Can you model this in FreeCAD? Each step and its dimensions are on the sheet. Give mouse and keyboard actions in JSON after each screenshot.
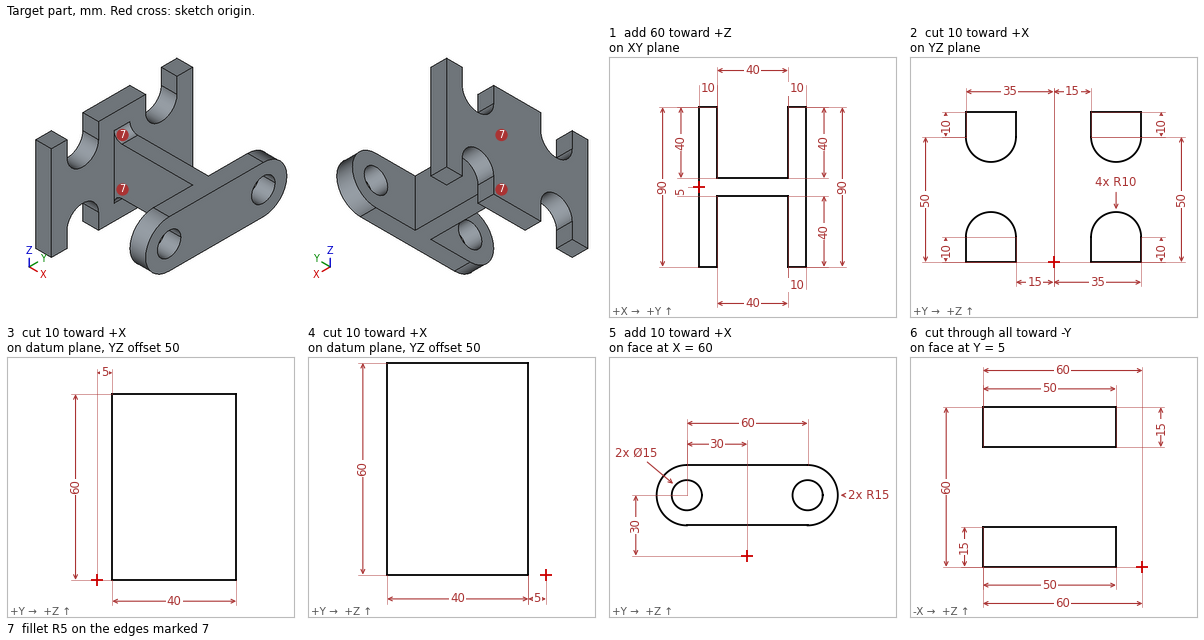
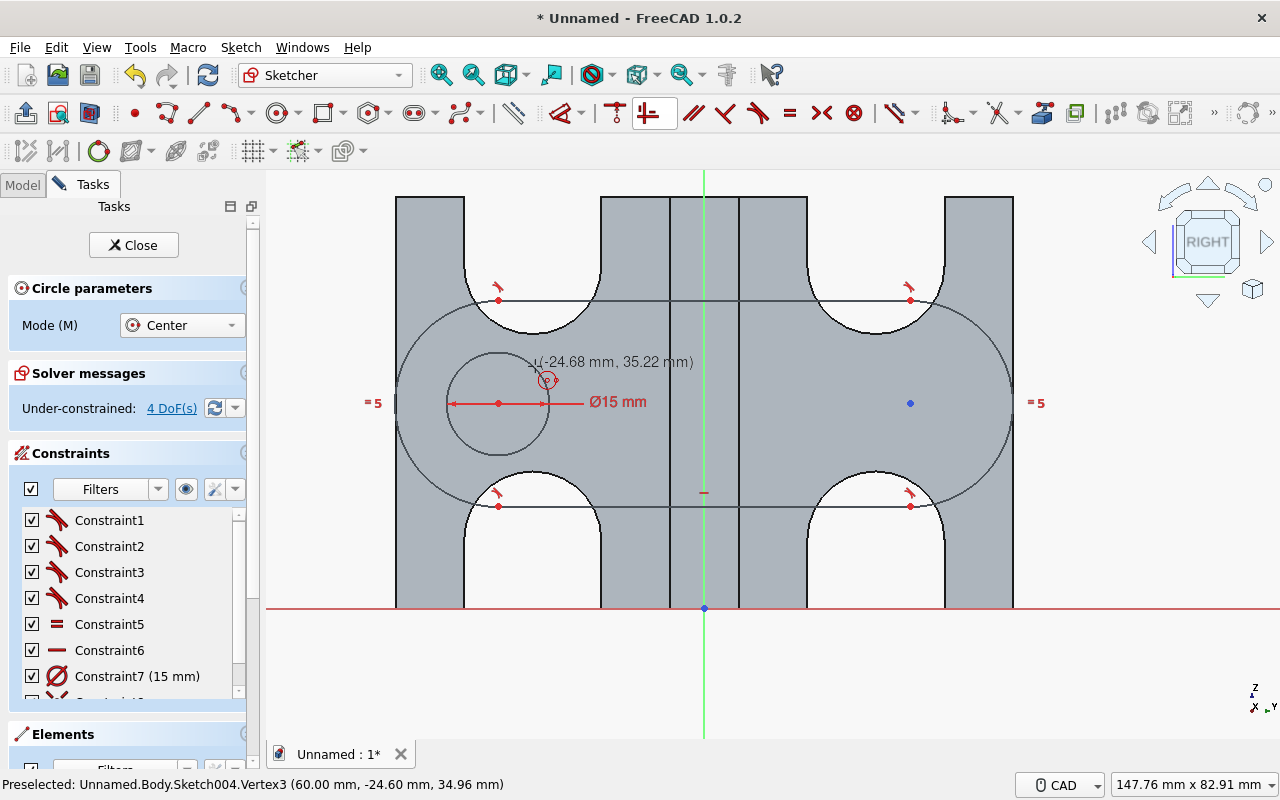
{"action": "left_click", "coordinate": [910, 404]}
{"action": "mouse_move", "coordinate": [947, 366]}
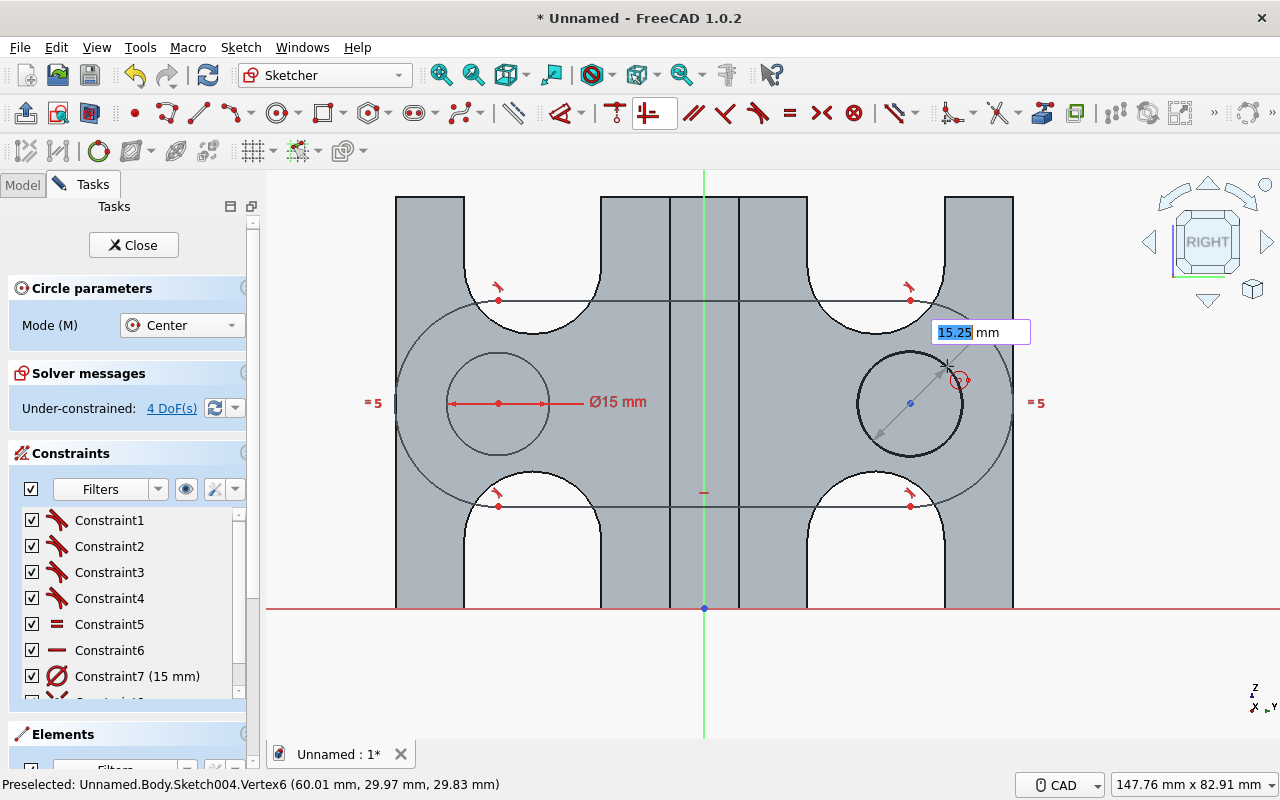
{"action": "type", "text": "15"}
{"action": "key", "text": "Return"}
{"action": "key", "text": "Escape"}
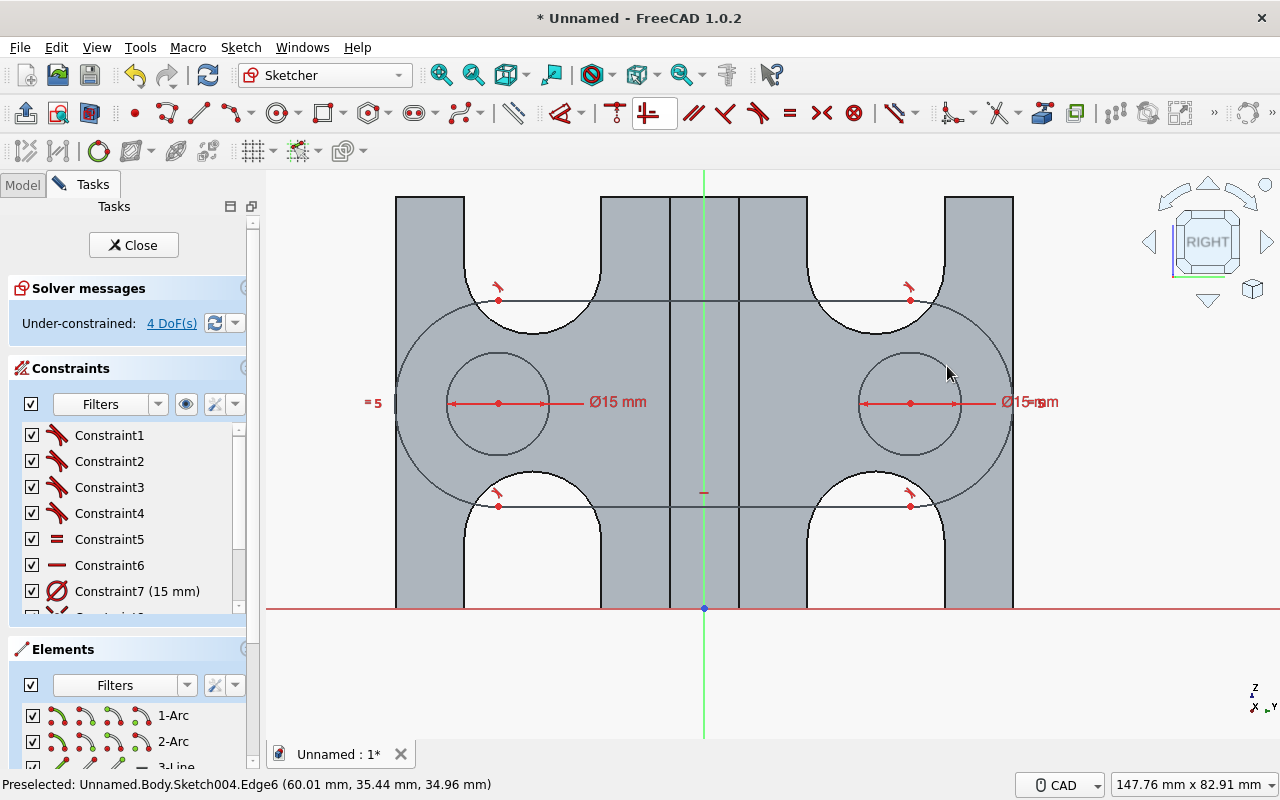
{"action": "left_click", "coordinate": [560, 114]}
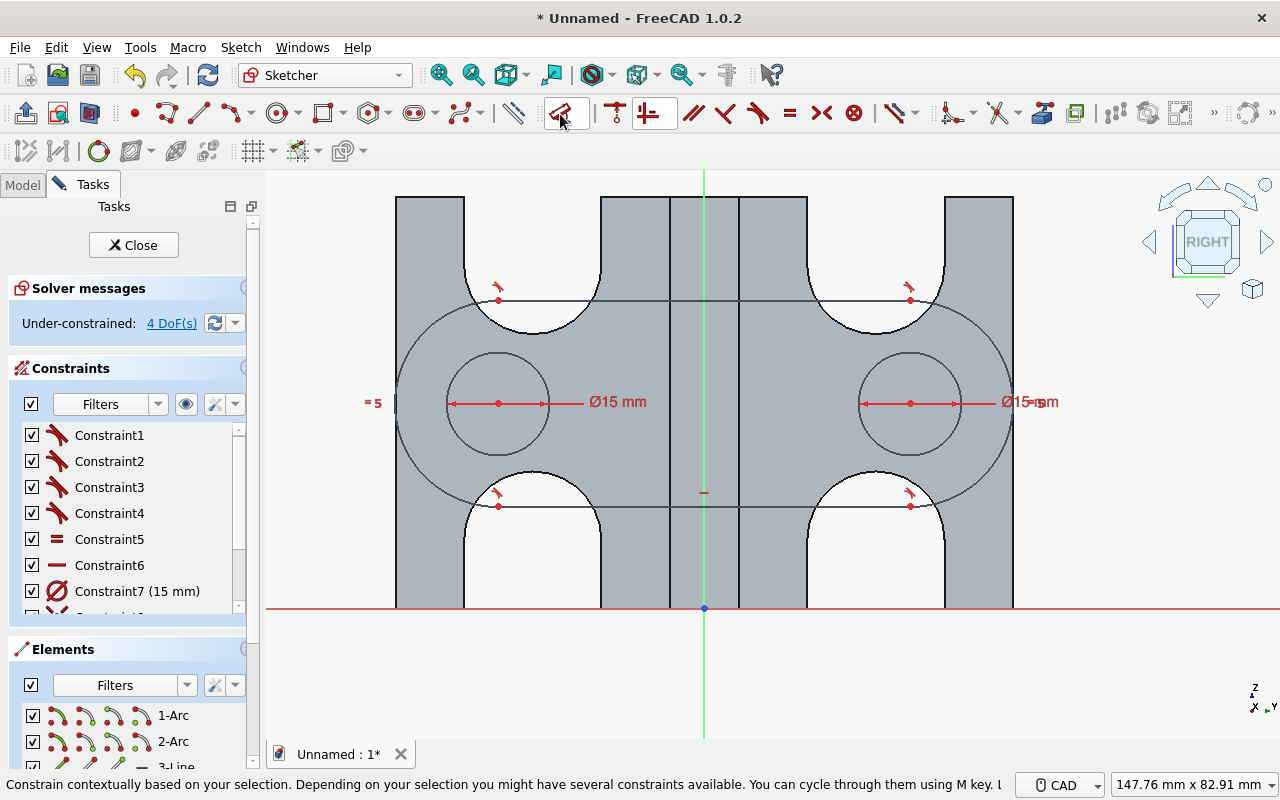
{"action": "left_click", "coordinate": [415, 343]}
{"action": "left_click", "coordinate": [389, 324]}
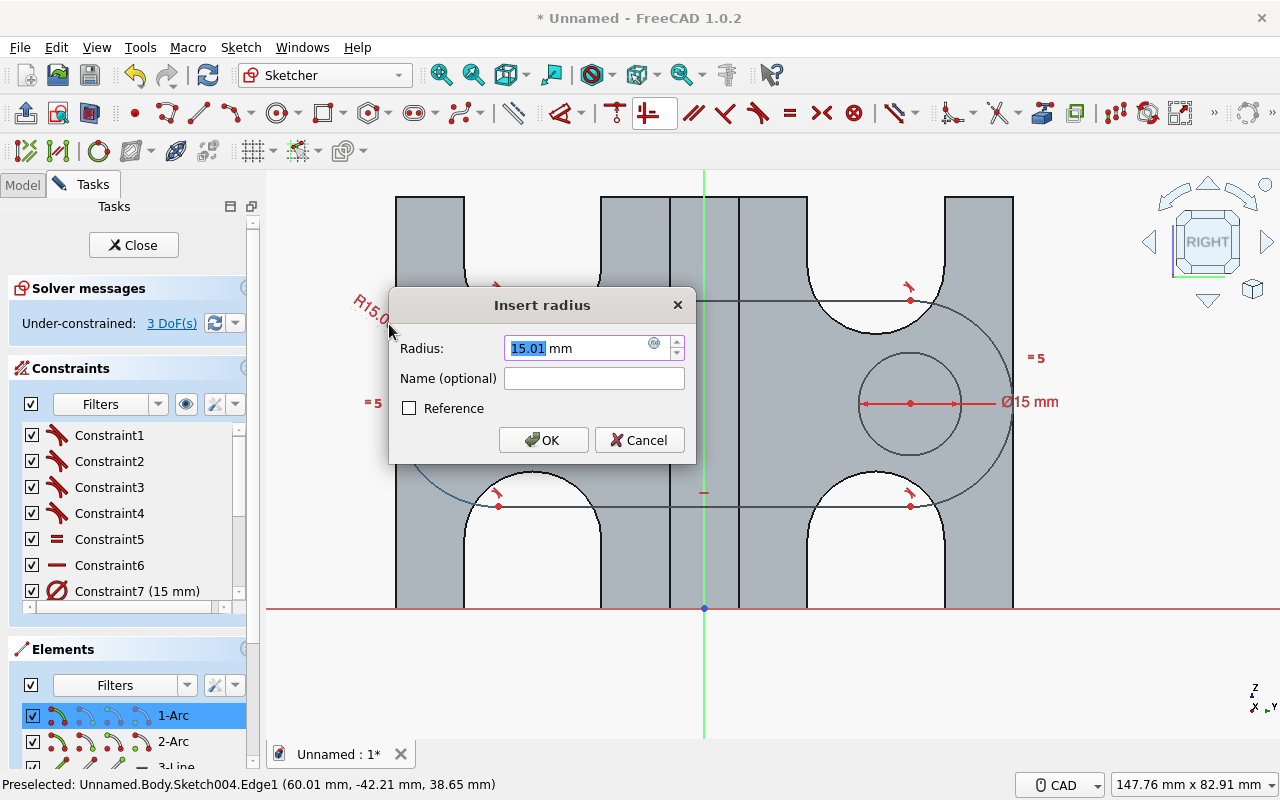
{"action": "type", "text": "15"}
{"action": "key", "text": "Return"}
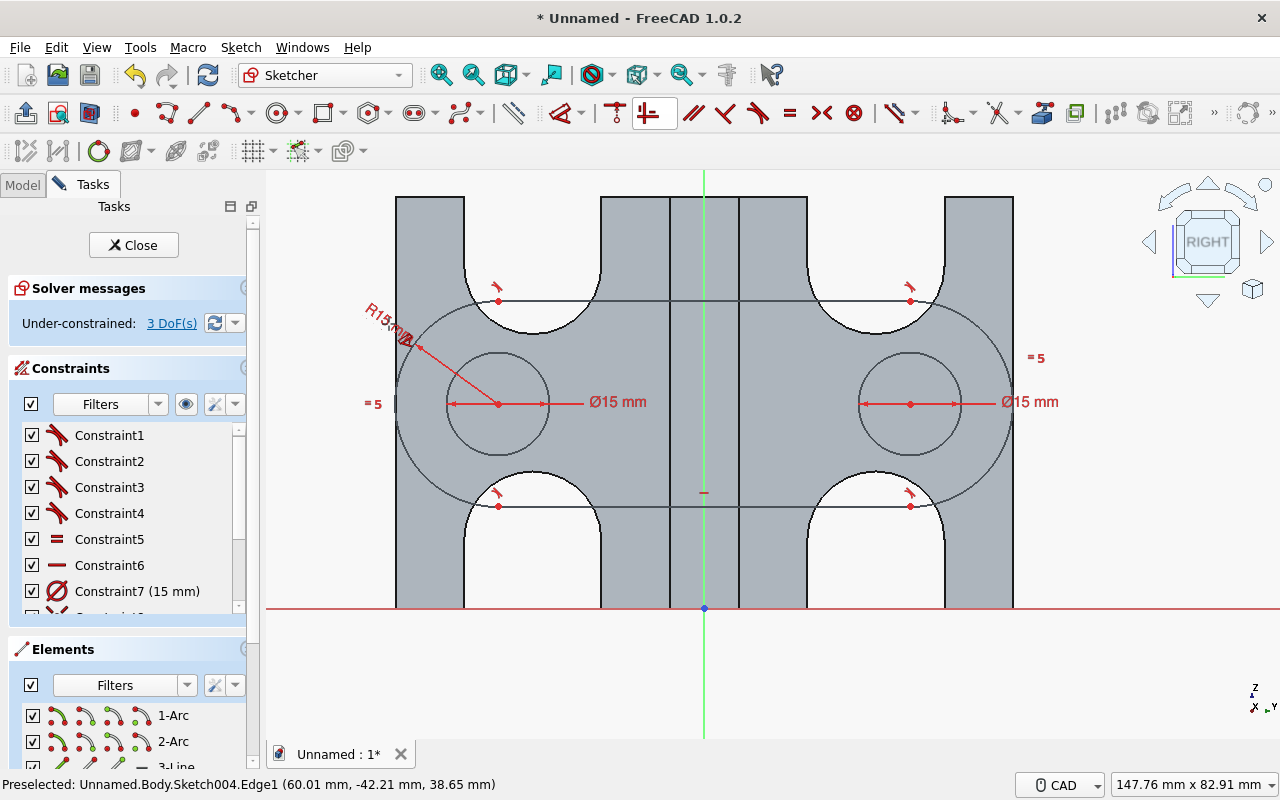
{"action": "left_click", "coordinate": [622, 301]}
{"action": "left_click", "coordinate": [609, 267]}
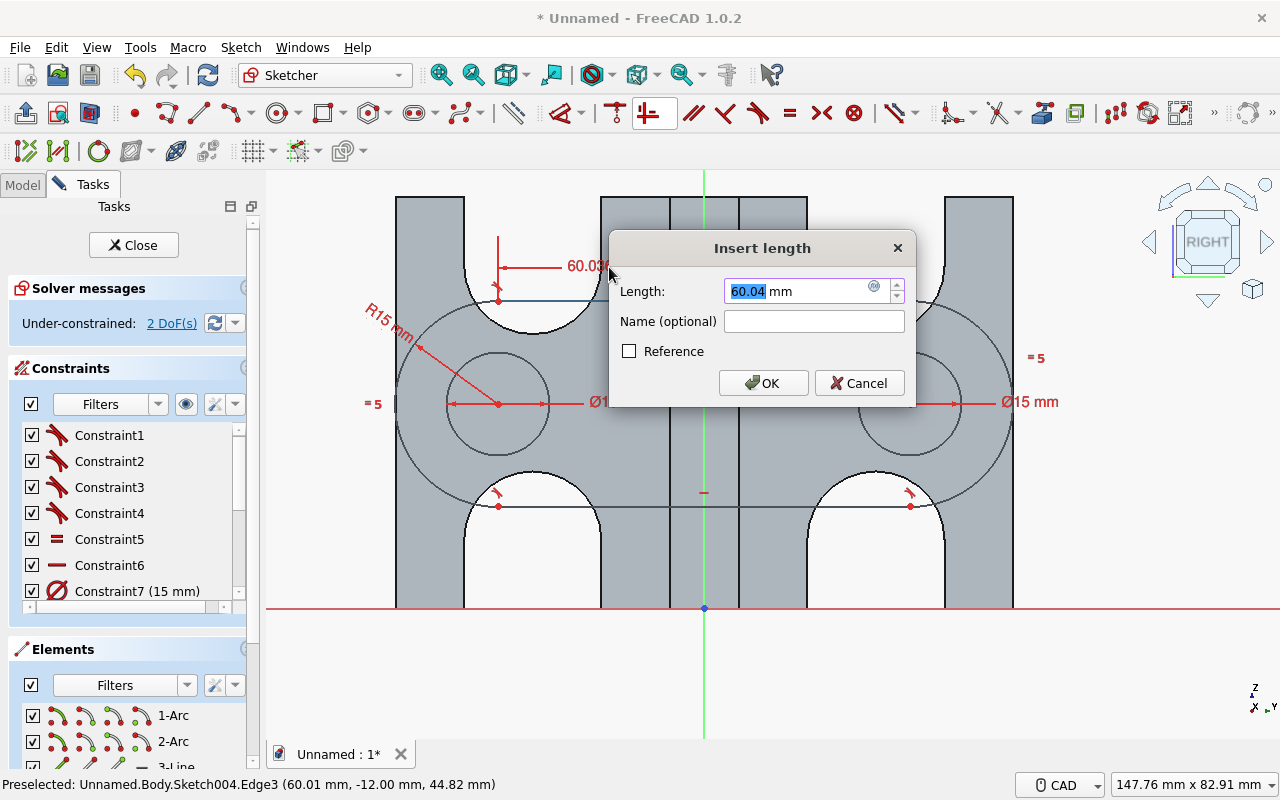
{"action": "type", "text": "60"}
{"action": "key", "text": "Return"}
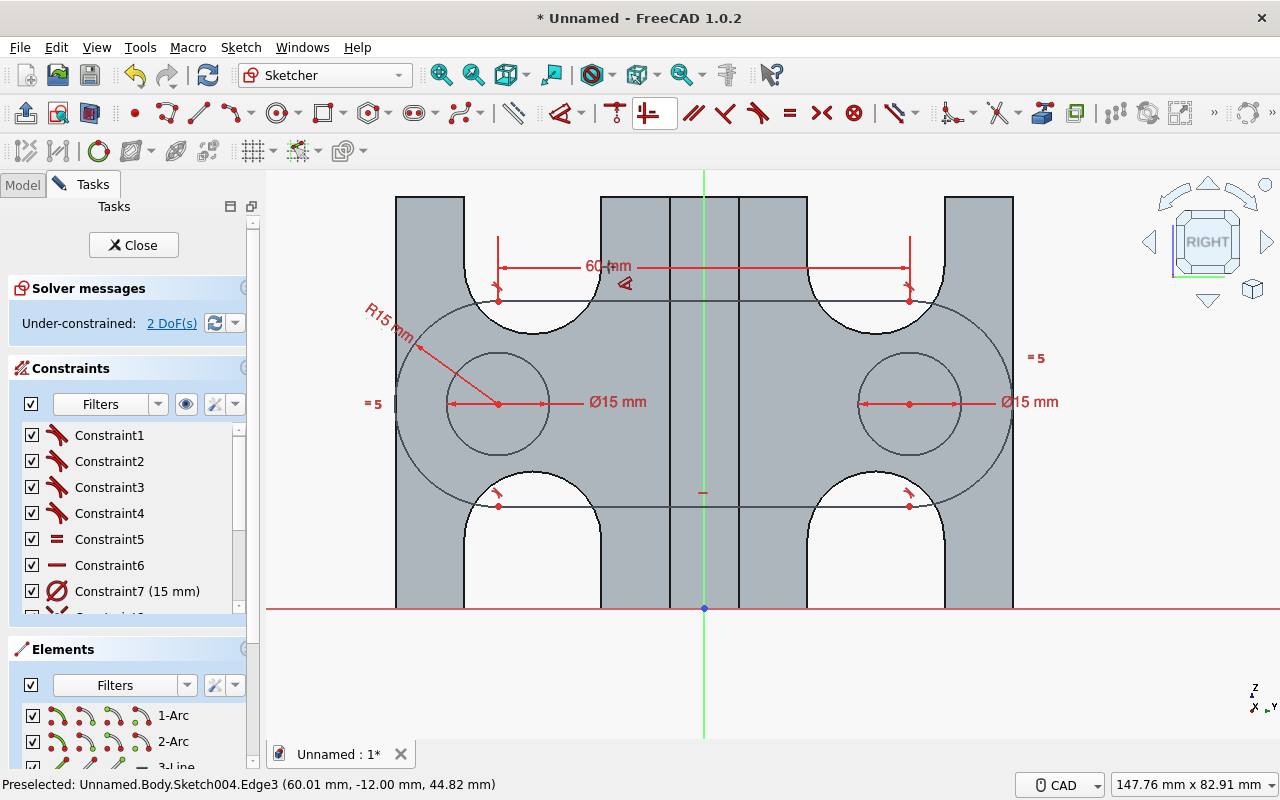
{"action": "left_click", "coordinate": [498, 404]}
{"action": "left_click", "coordinate": [601, 643]}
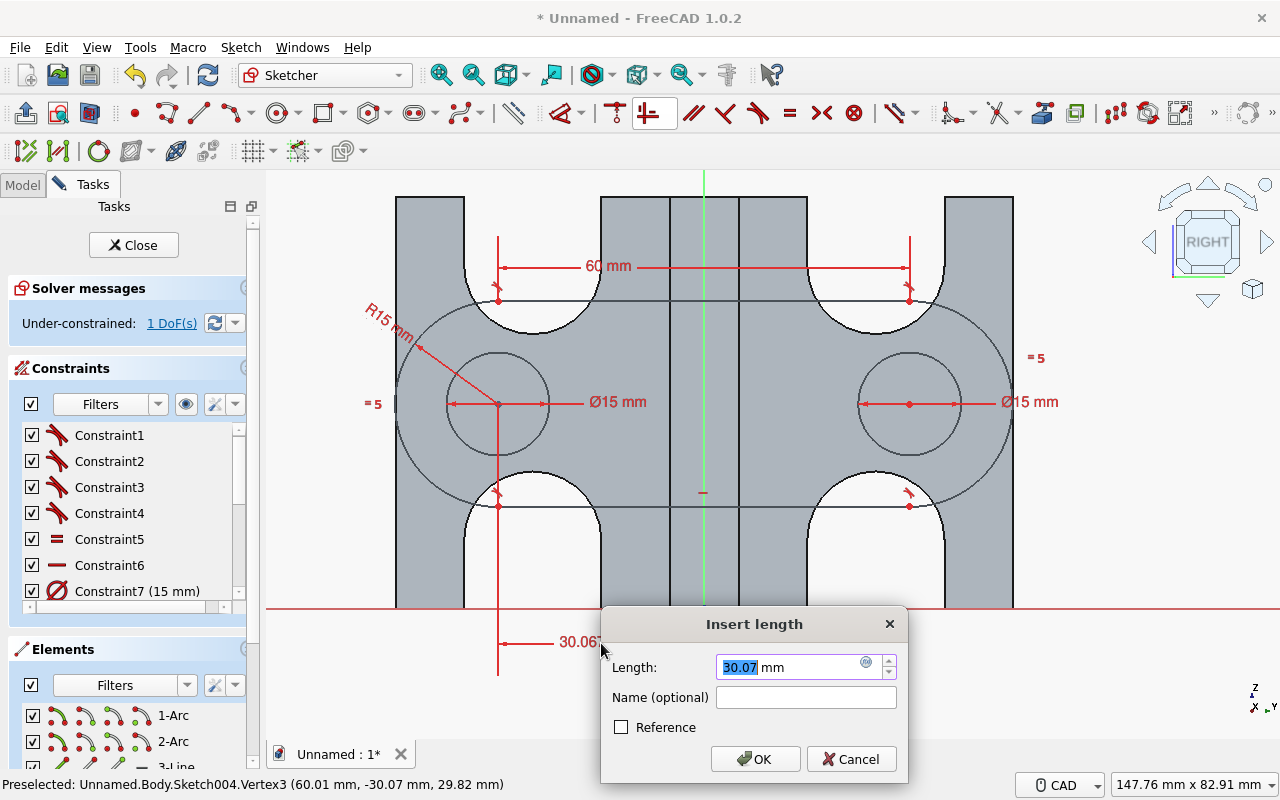
{"action": "type", "text": "30"}
{"action": "key", "text": "Return"}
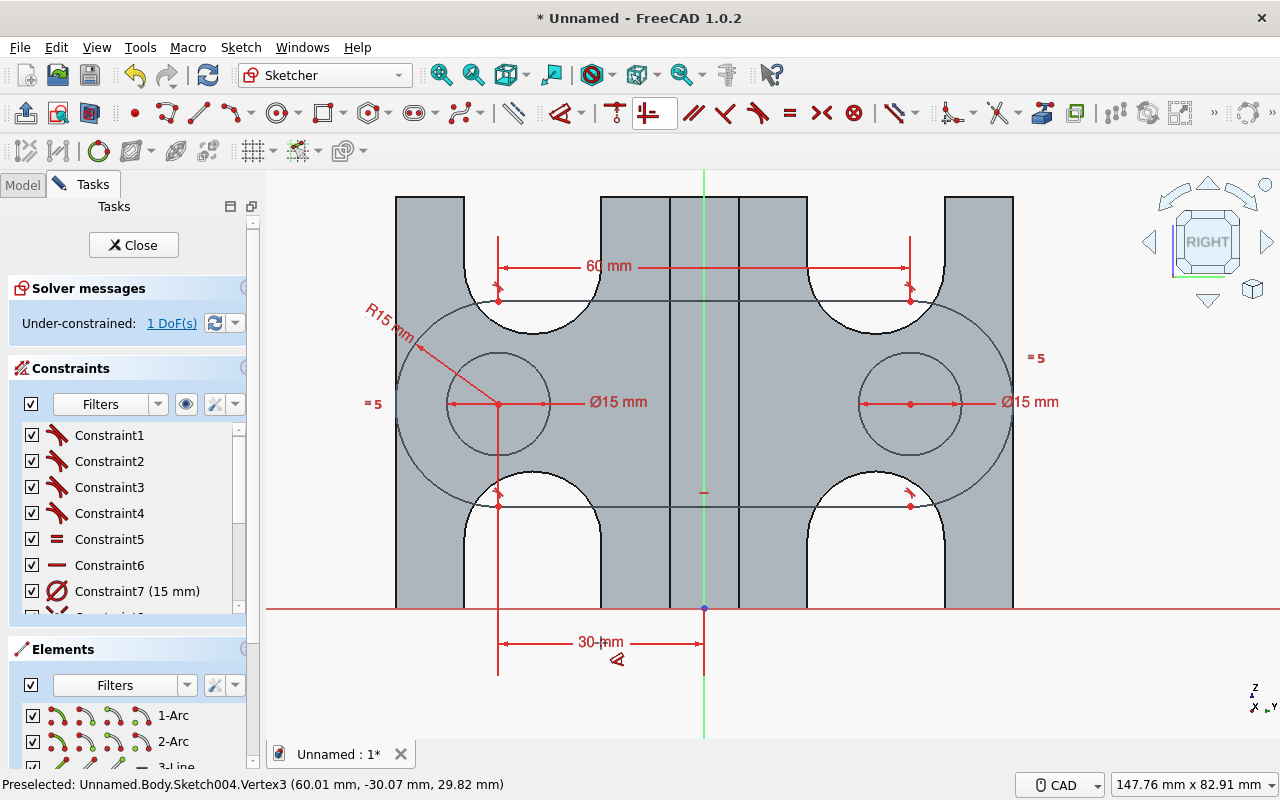
{"action": "left_click", "coordinate": [498, 404]}
{"action": "left_click", "coordinate": [464, 459]}